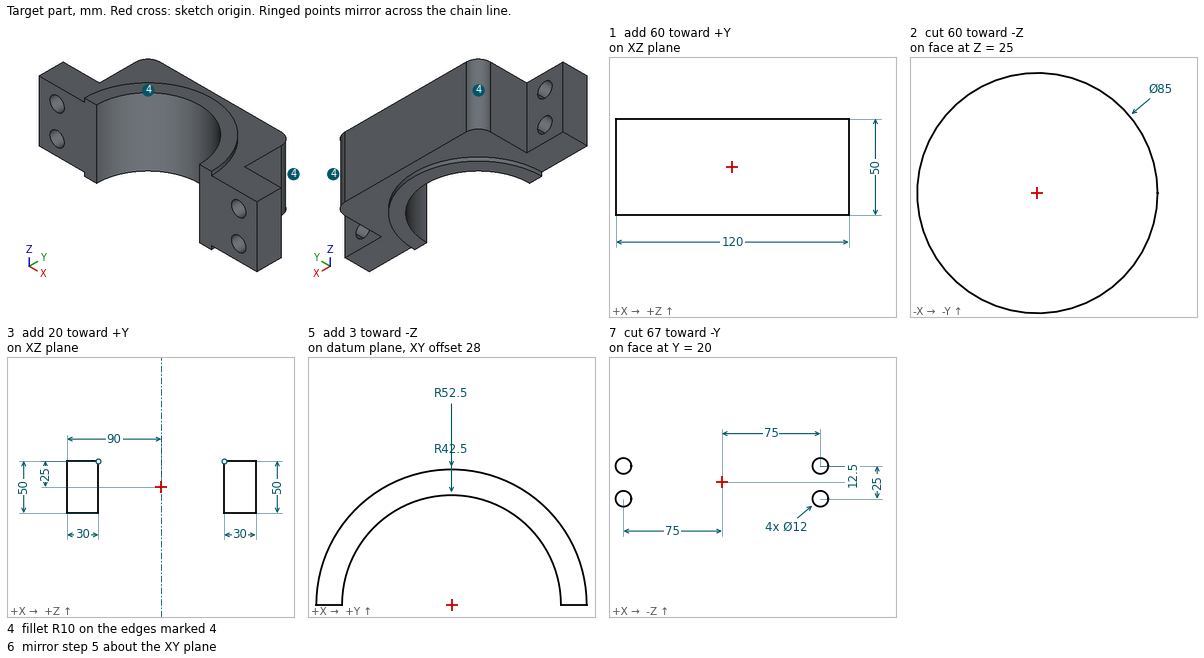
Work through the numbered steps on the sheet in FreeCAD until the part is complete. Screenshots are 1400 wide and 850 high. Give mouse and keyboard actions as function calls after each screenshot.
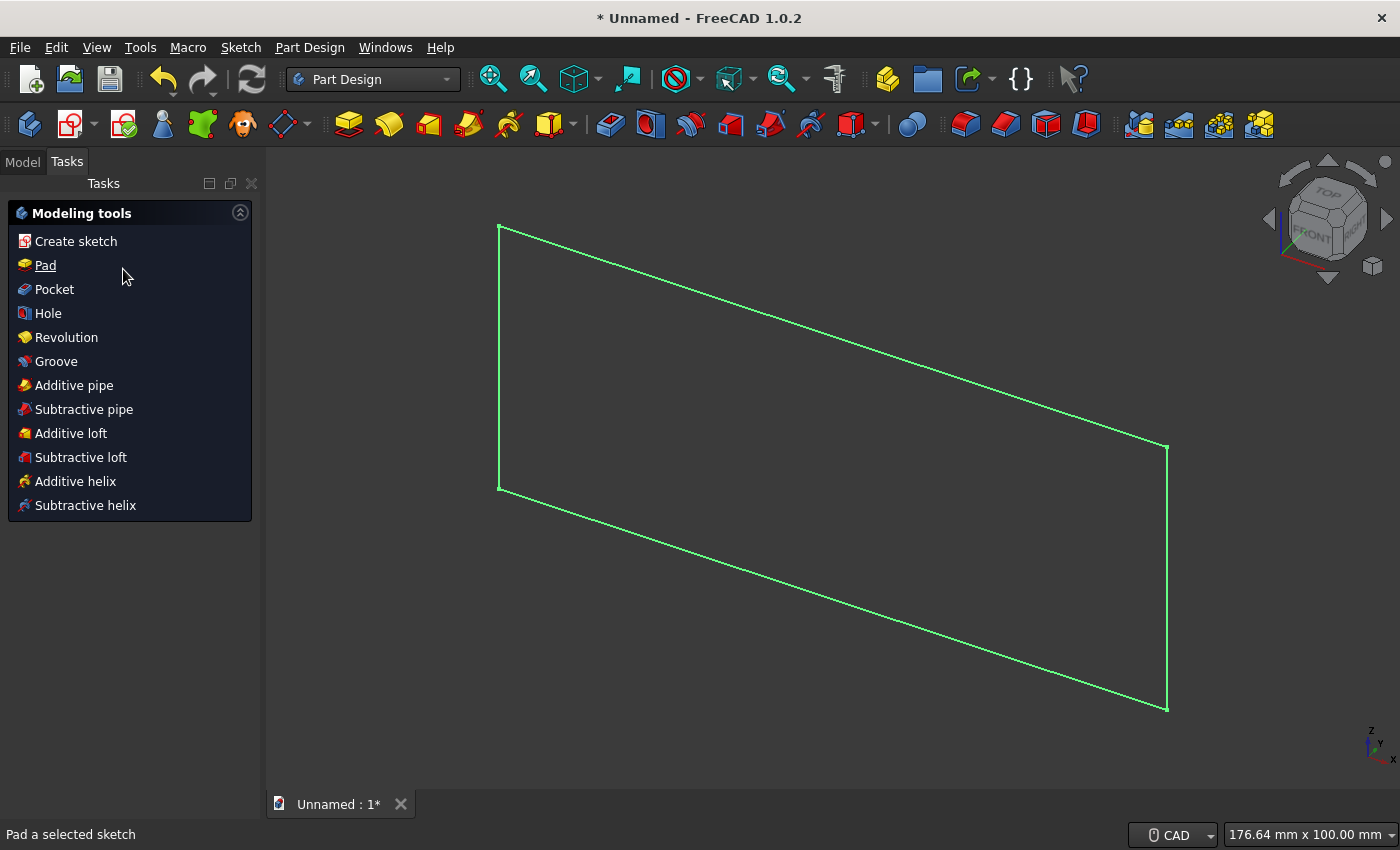
click(350, 124)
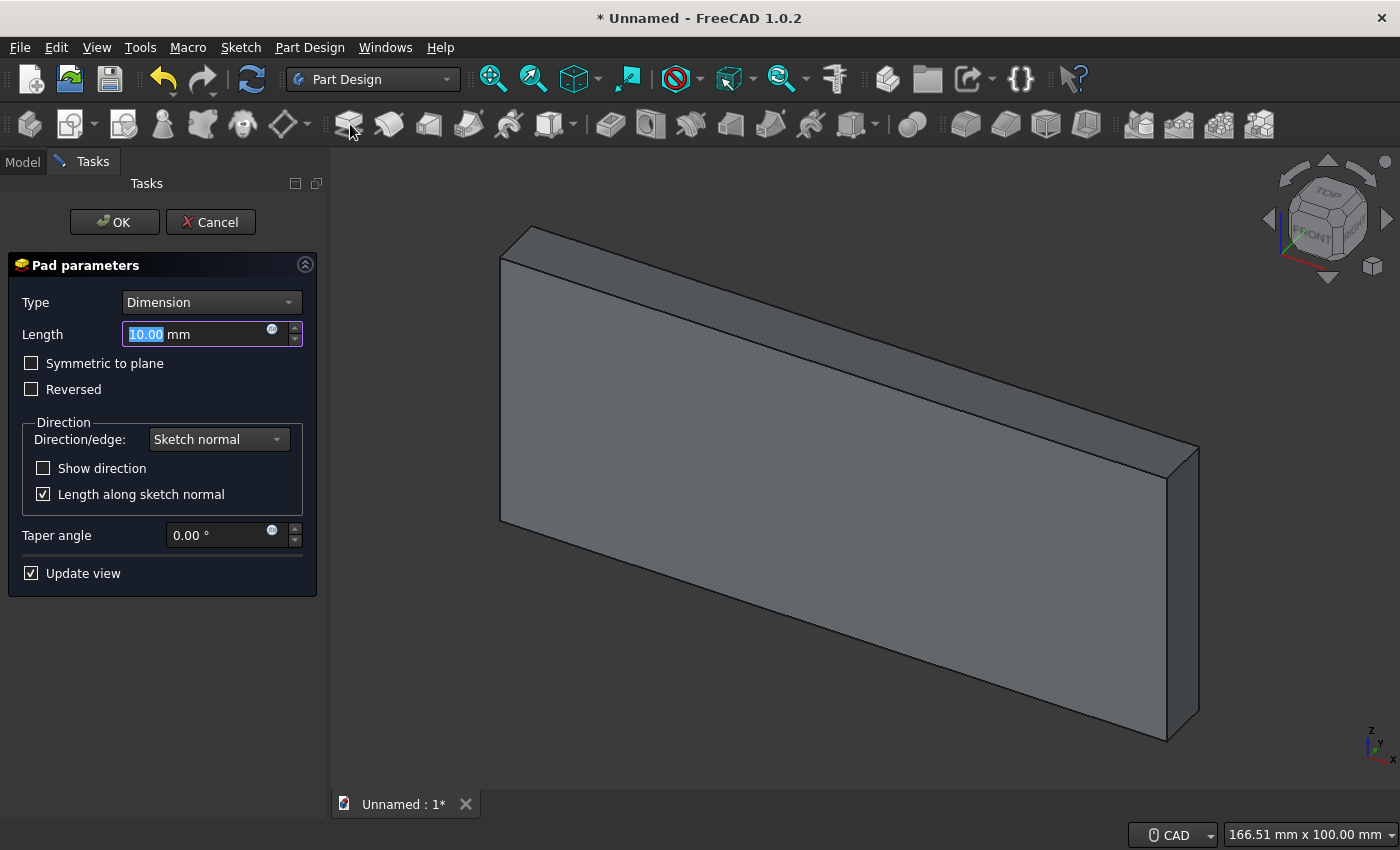
text(60)
key(Tab)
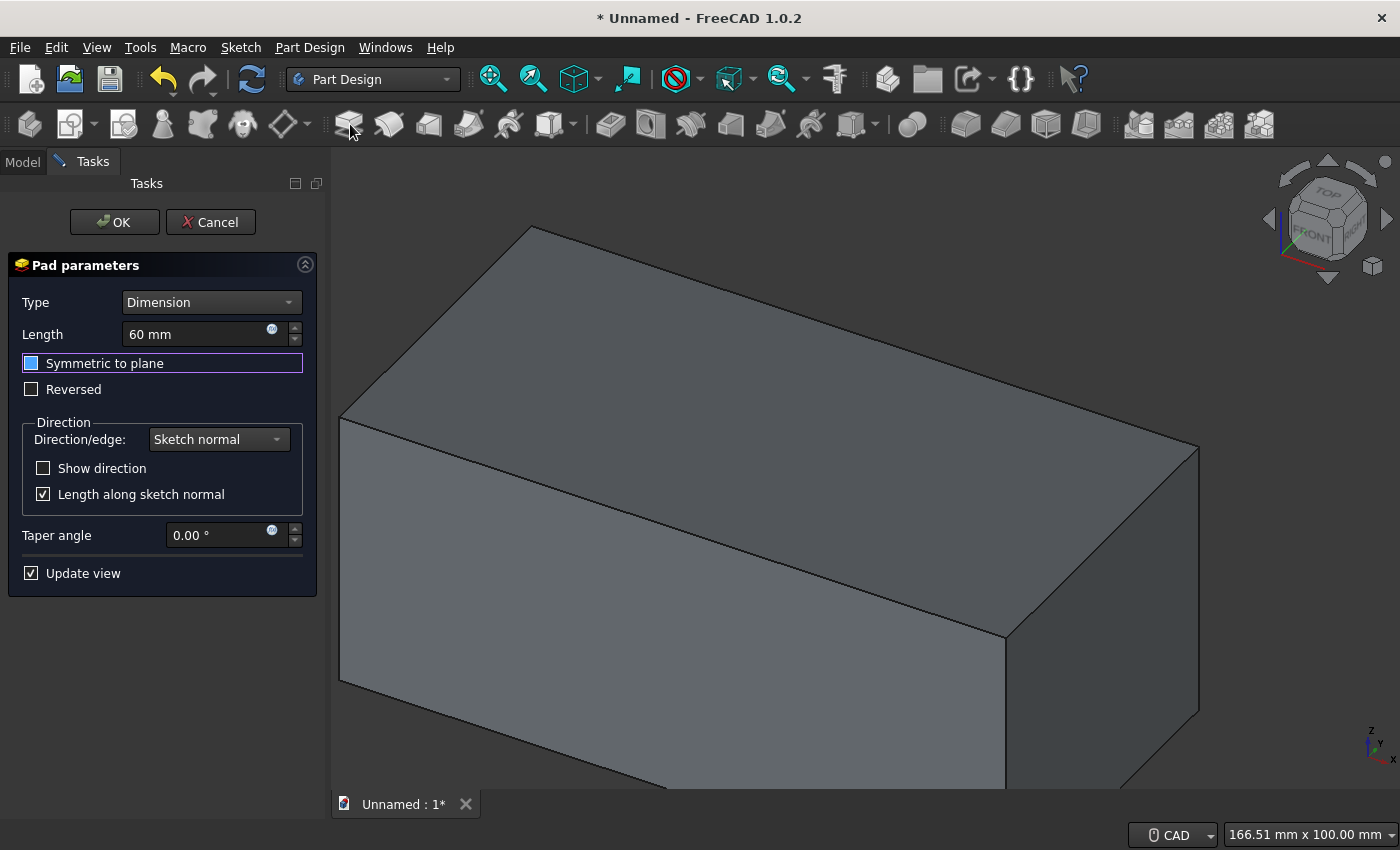
click(30, 389)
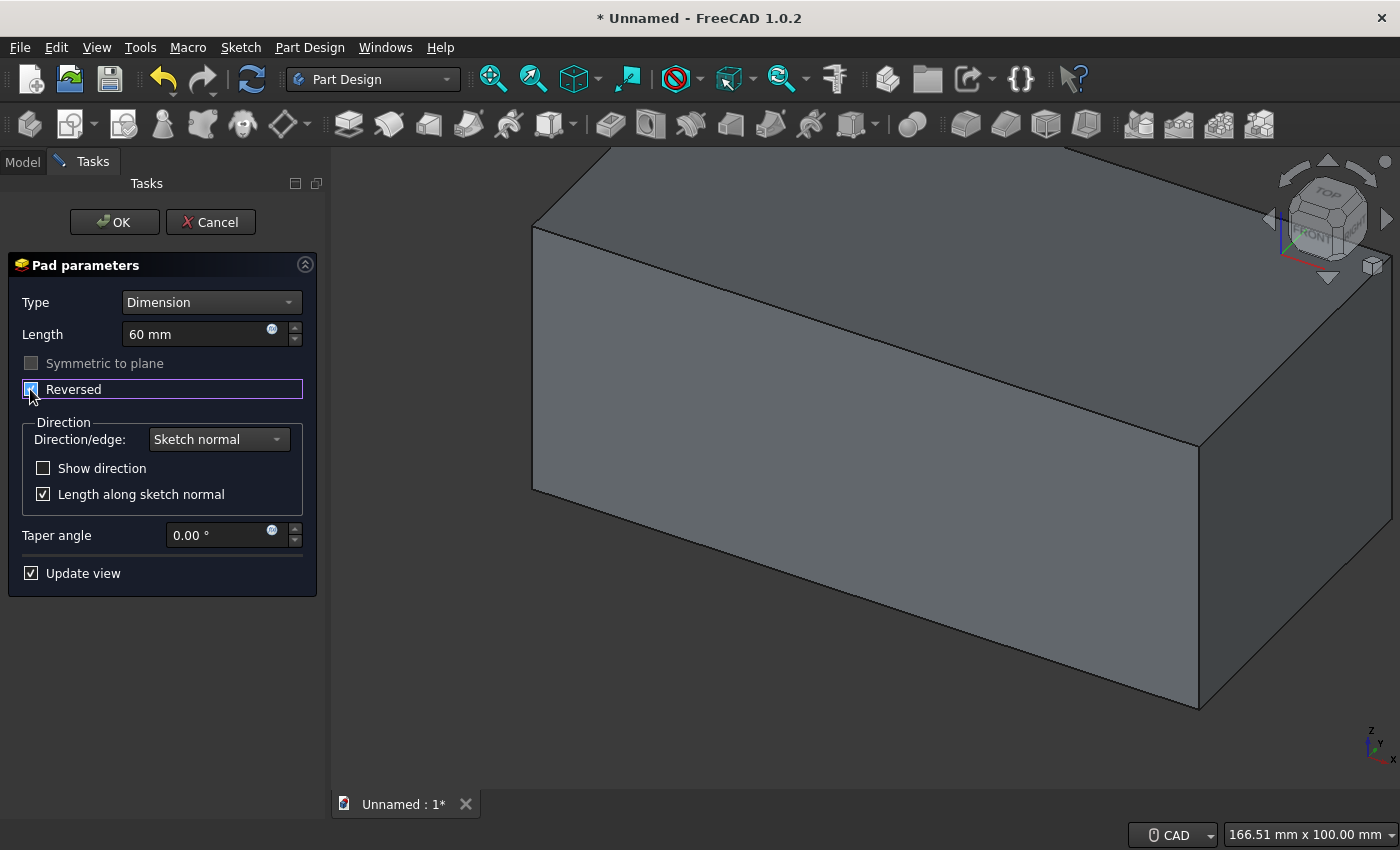
click(115, 222)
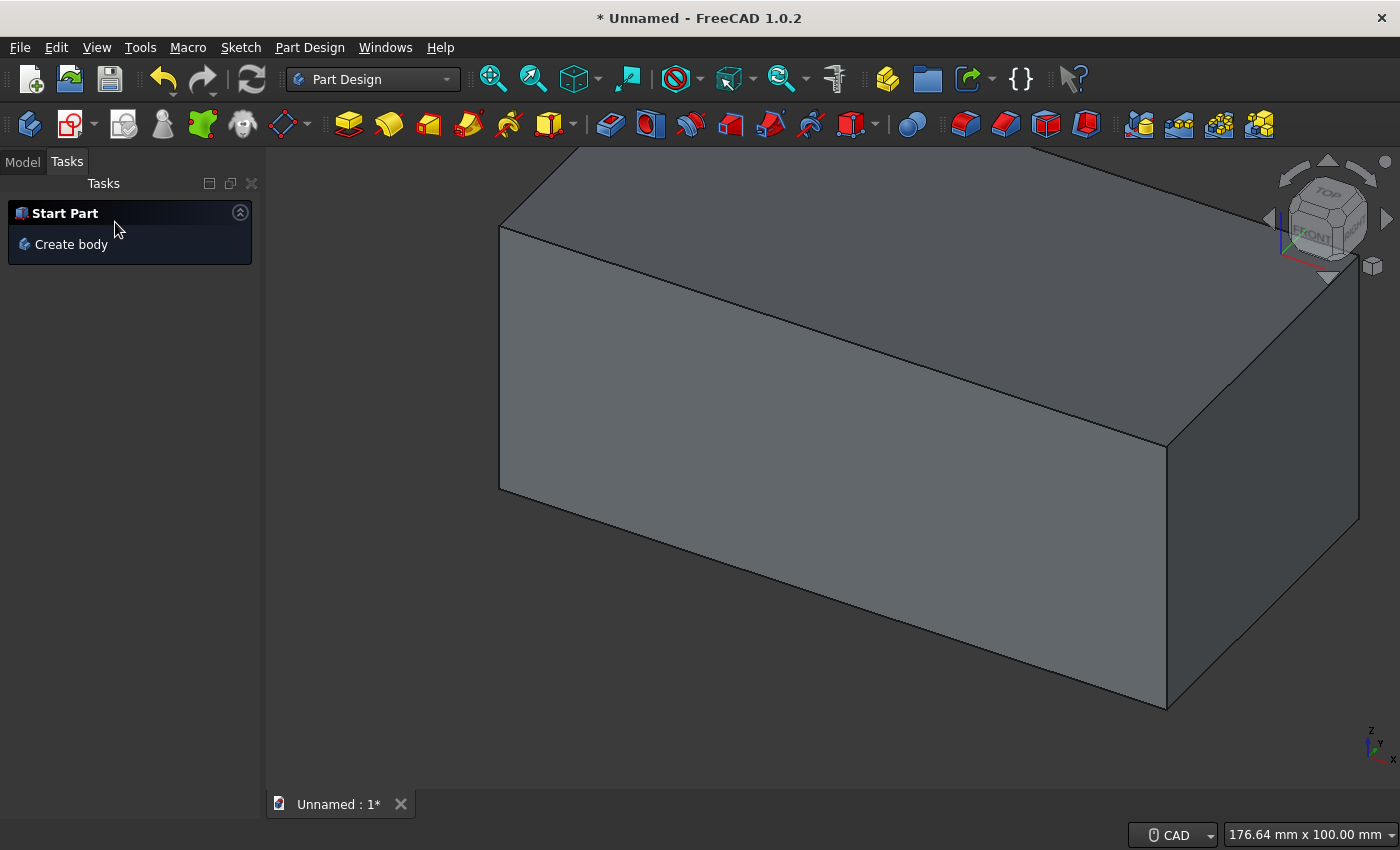
click(494, 80)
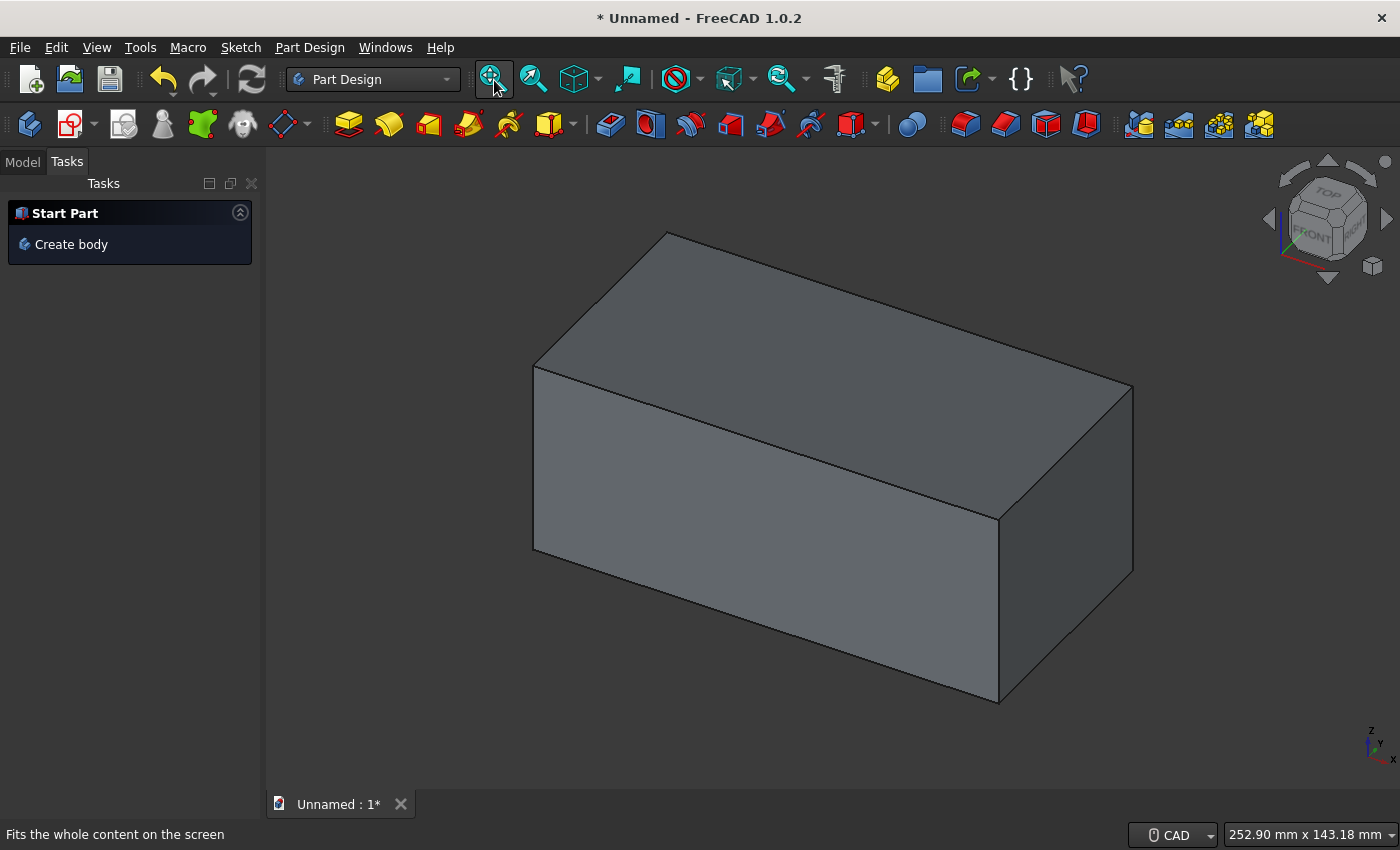
click(900, 397)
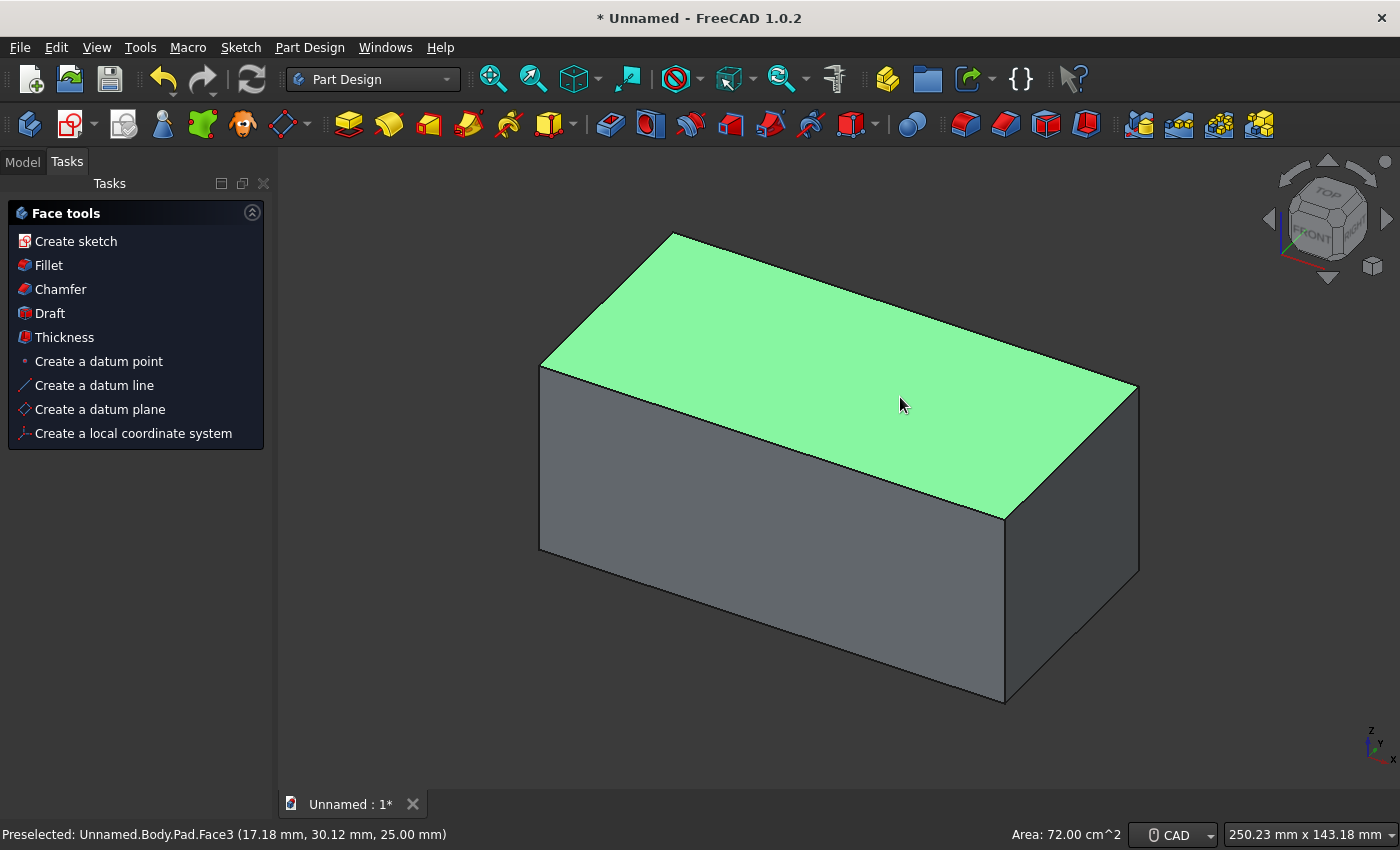
click(70, 124)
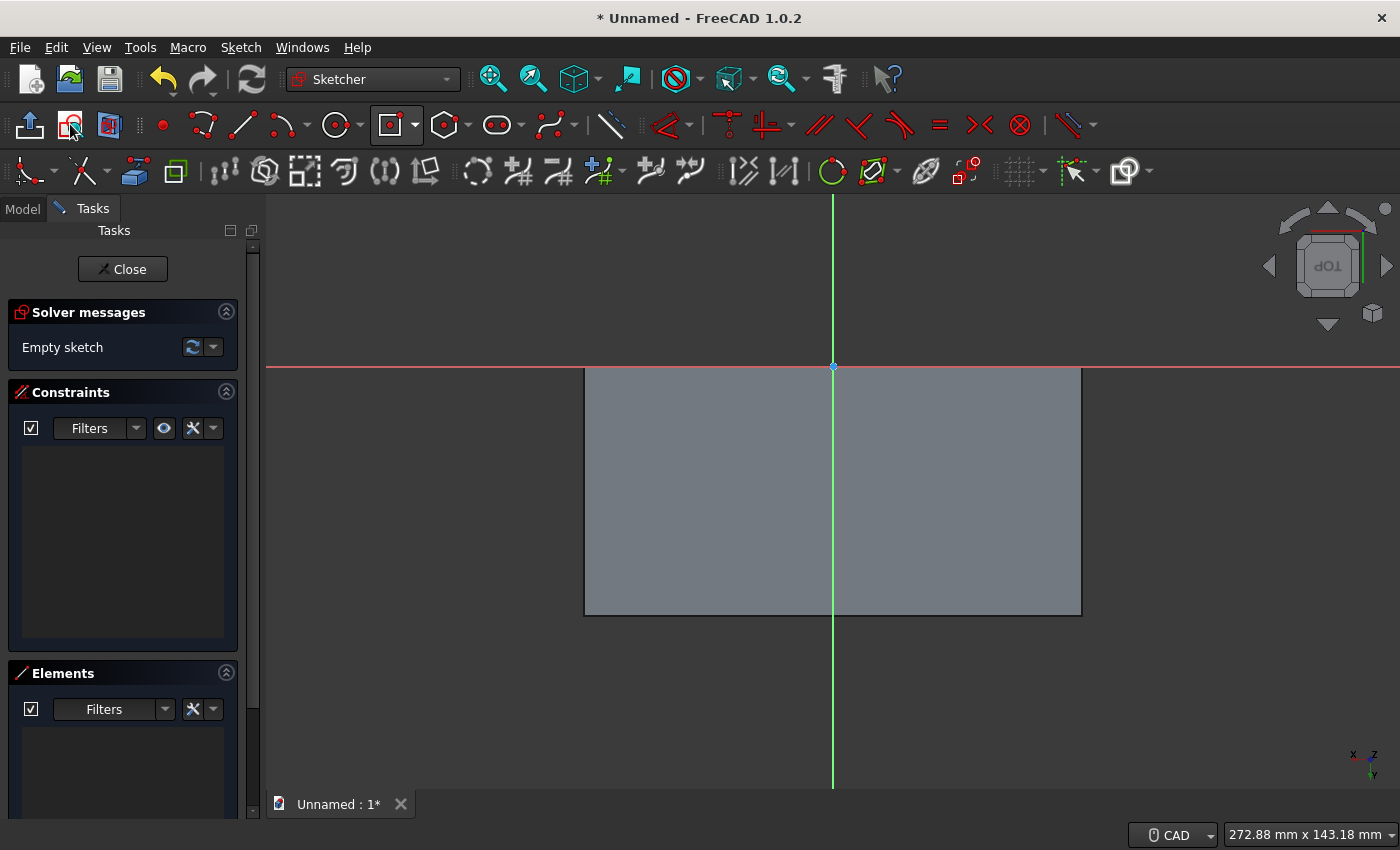
scroll(455, 761, down, 1)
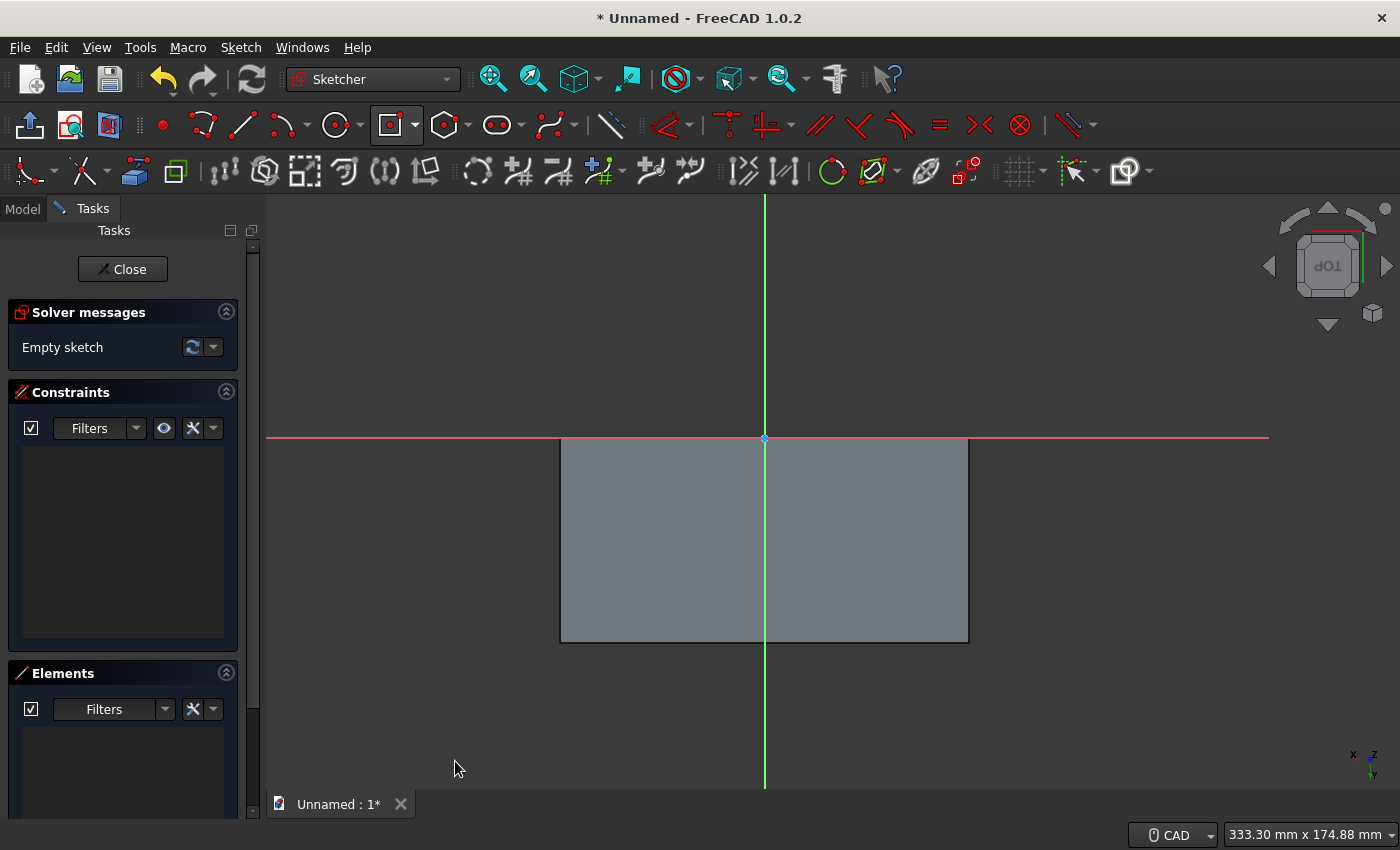
click(336, 126)